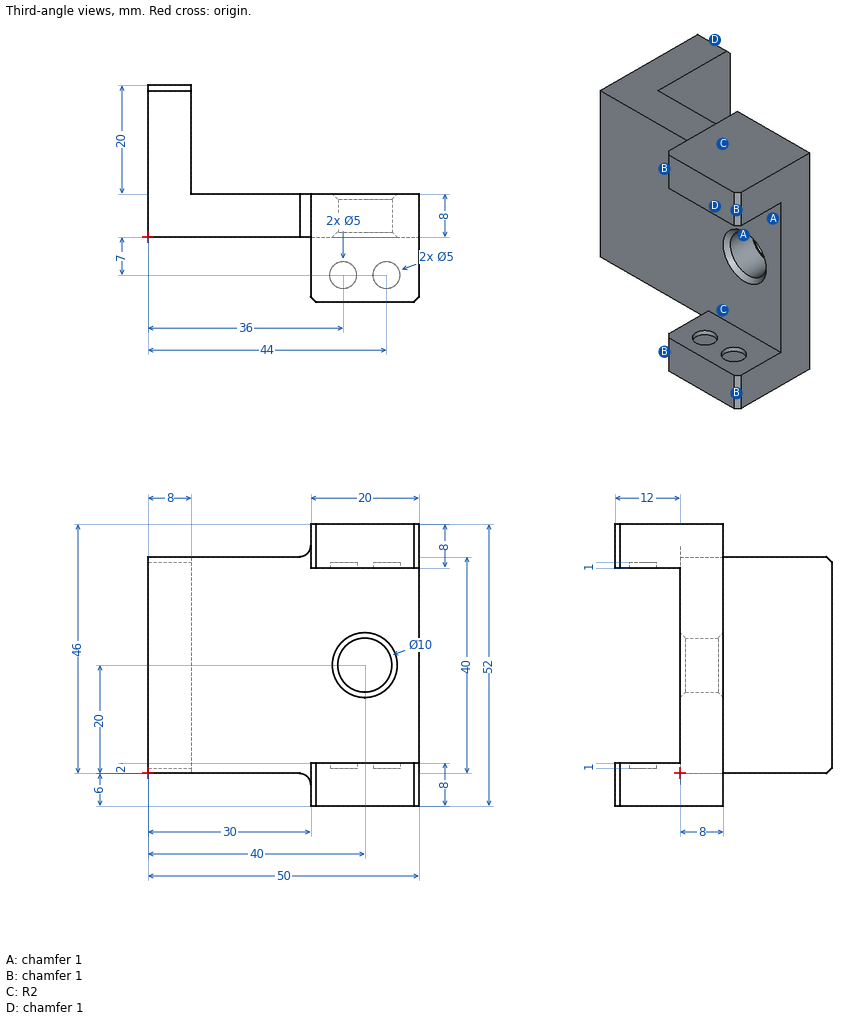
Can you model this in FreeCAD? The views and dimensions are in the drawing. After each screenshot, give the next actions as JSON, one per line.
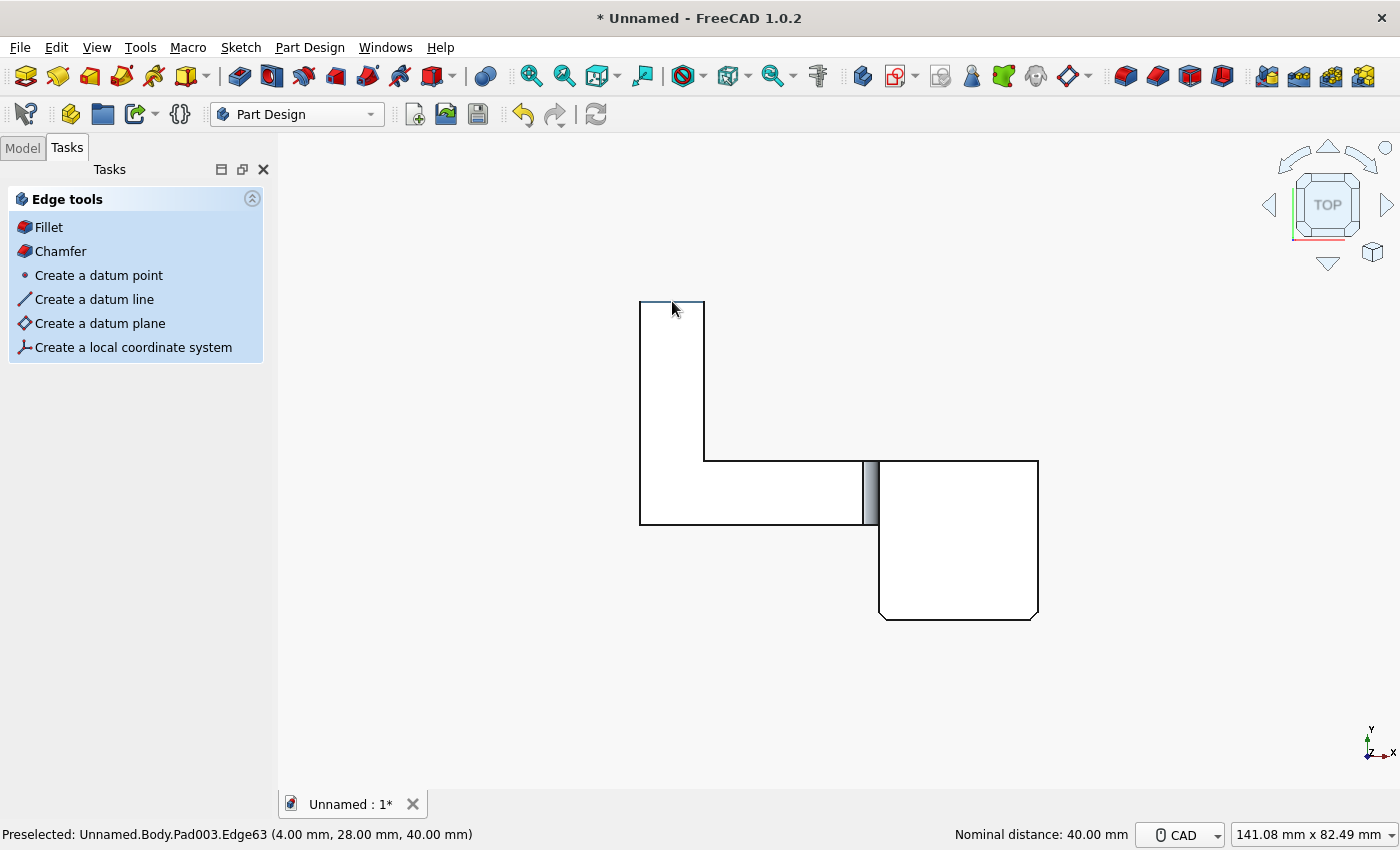
{"action": "left_click", "coordinate": [1158, 76]}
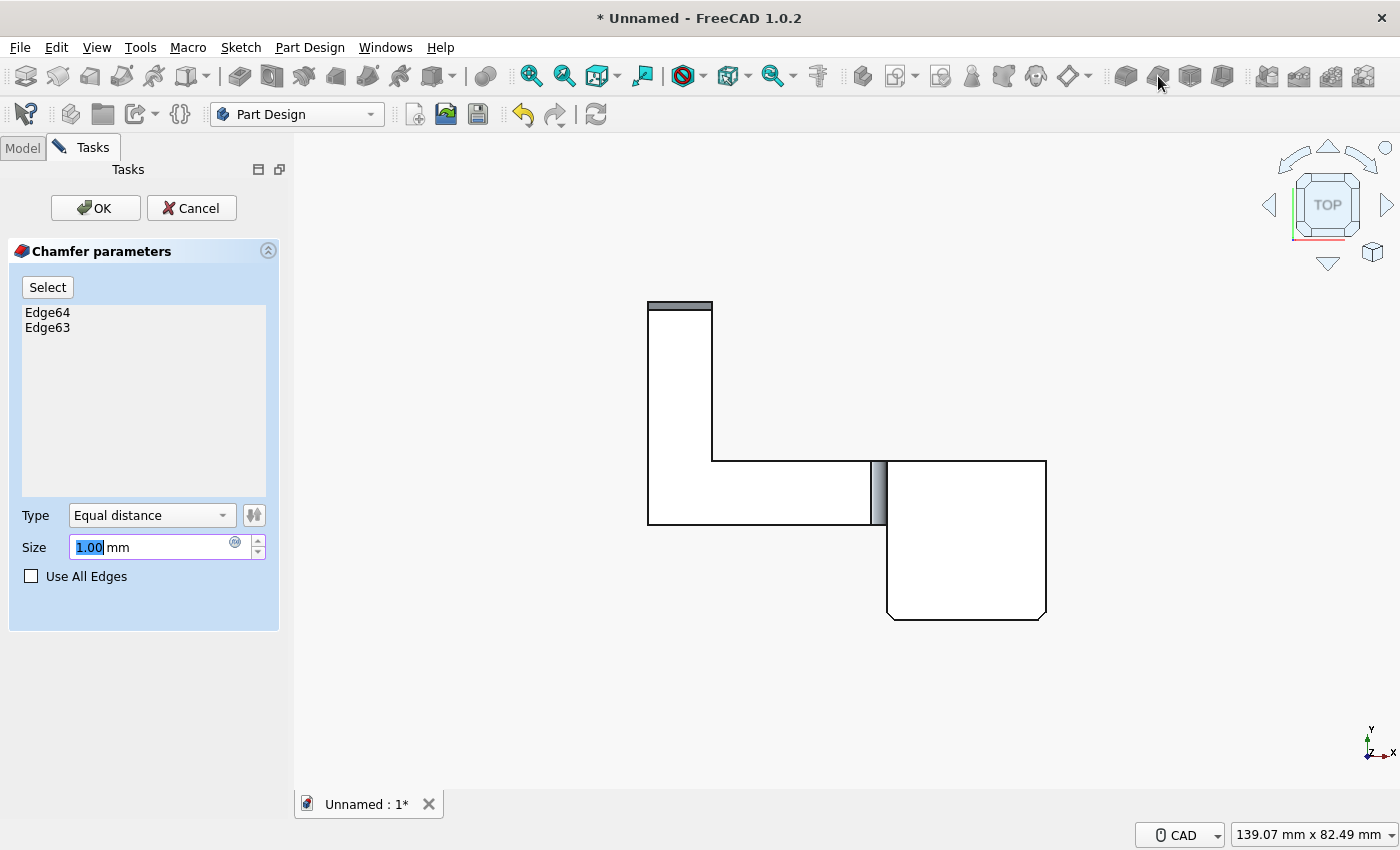
{"action": "type", "text": "1"}
{"action": "key", "text": "Tab"}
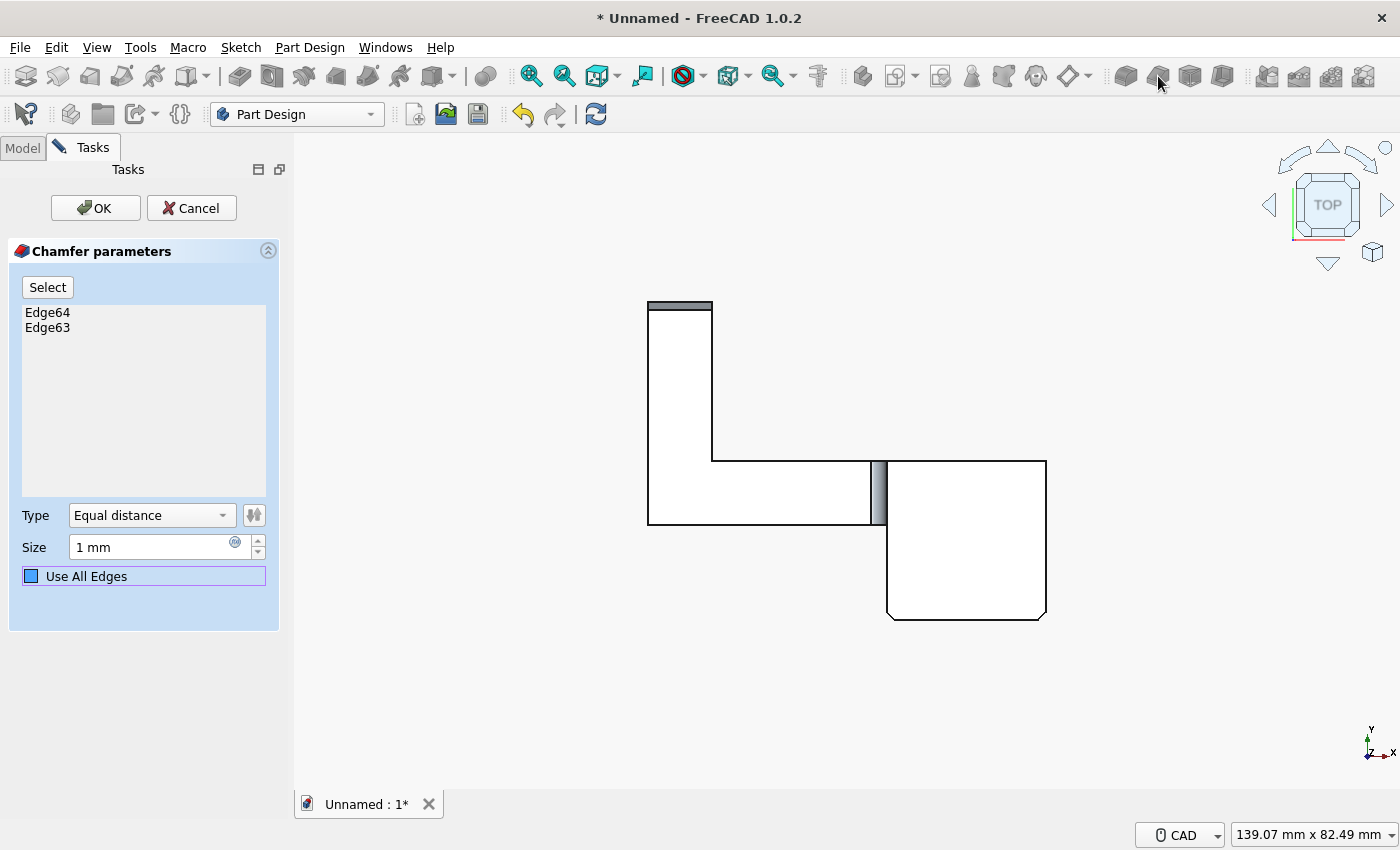
{"action": "left_click", "coordinate": [96, 208]}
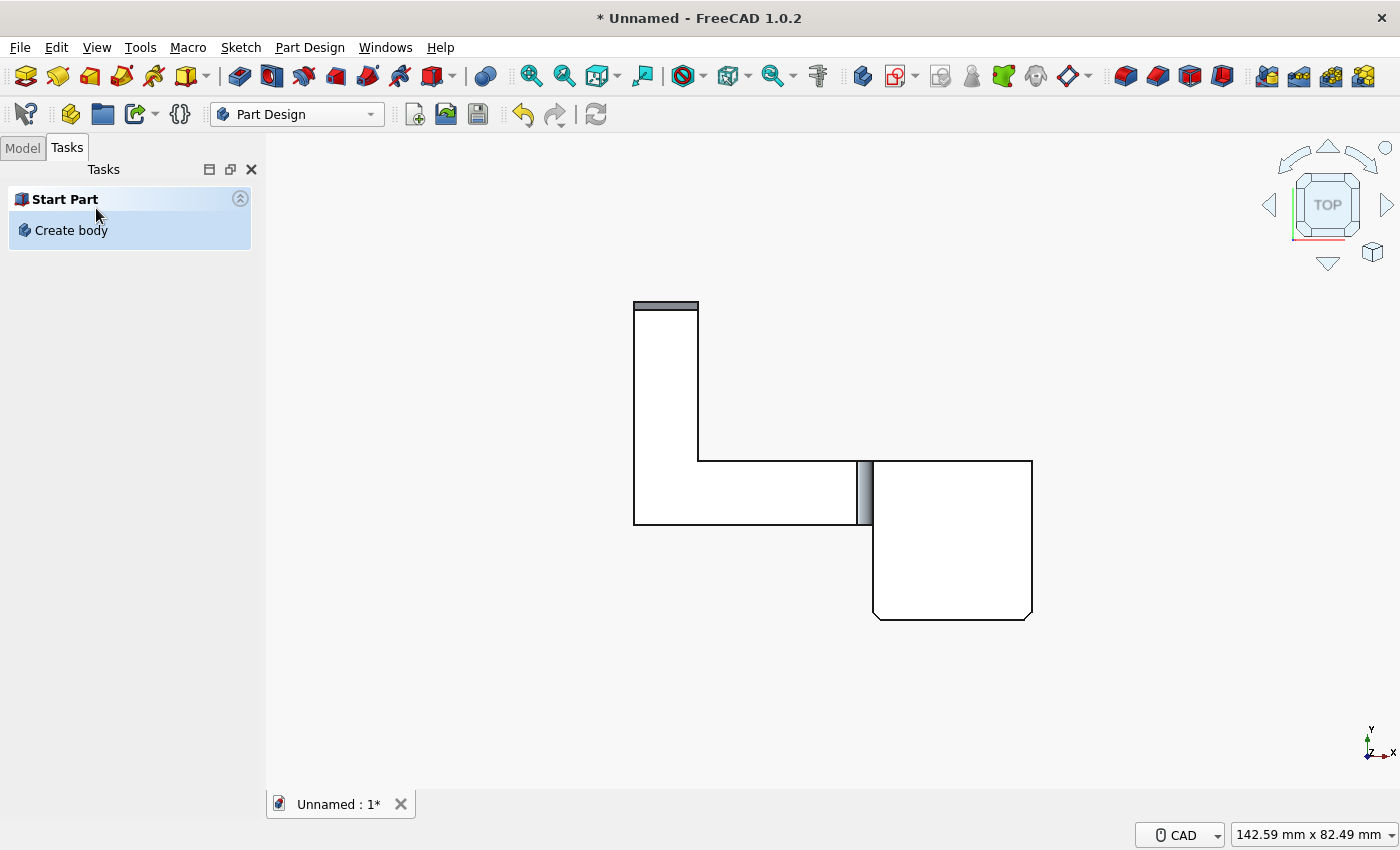
{"action": "left_click", "coordinate": [23, 147]}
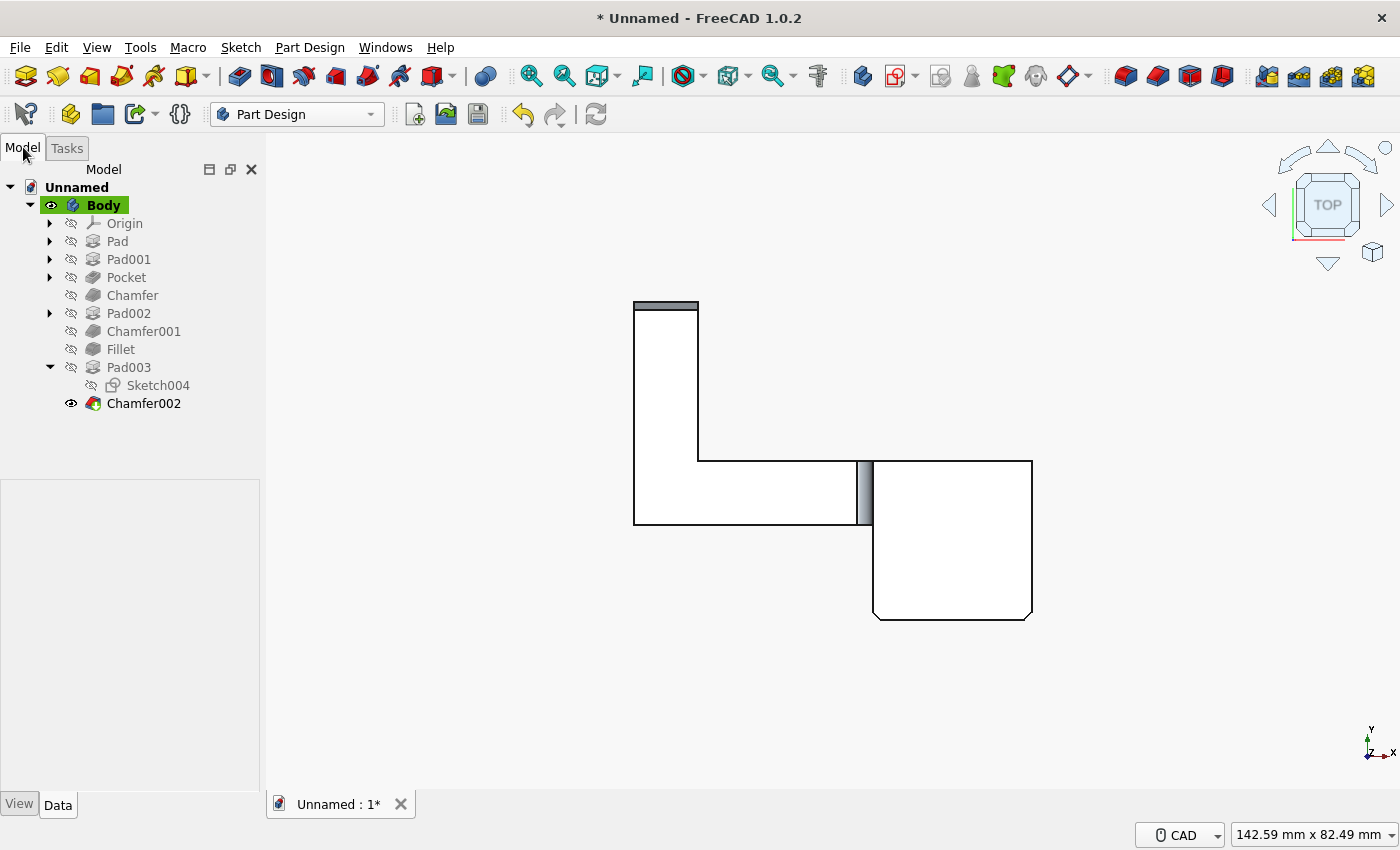
{"action": "left_click", "coordinate": [50, 223]}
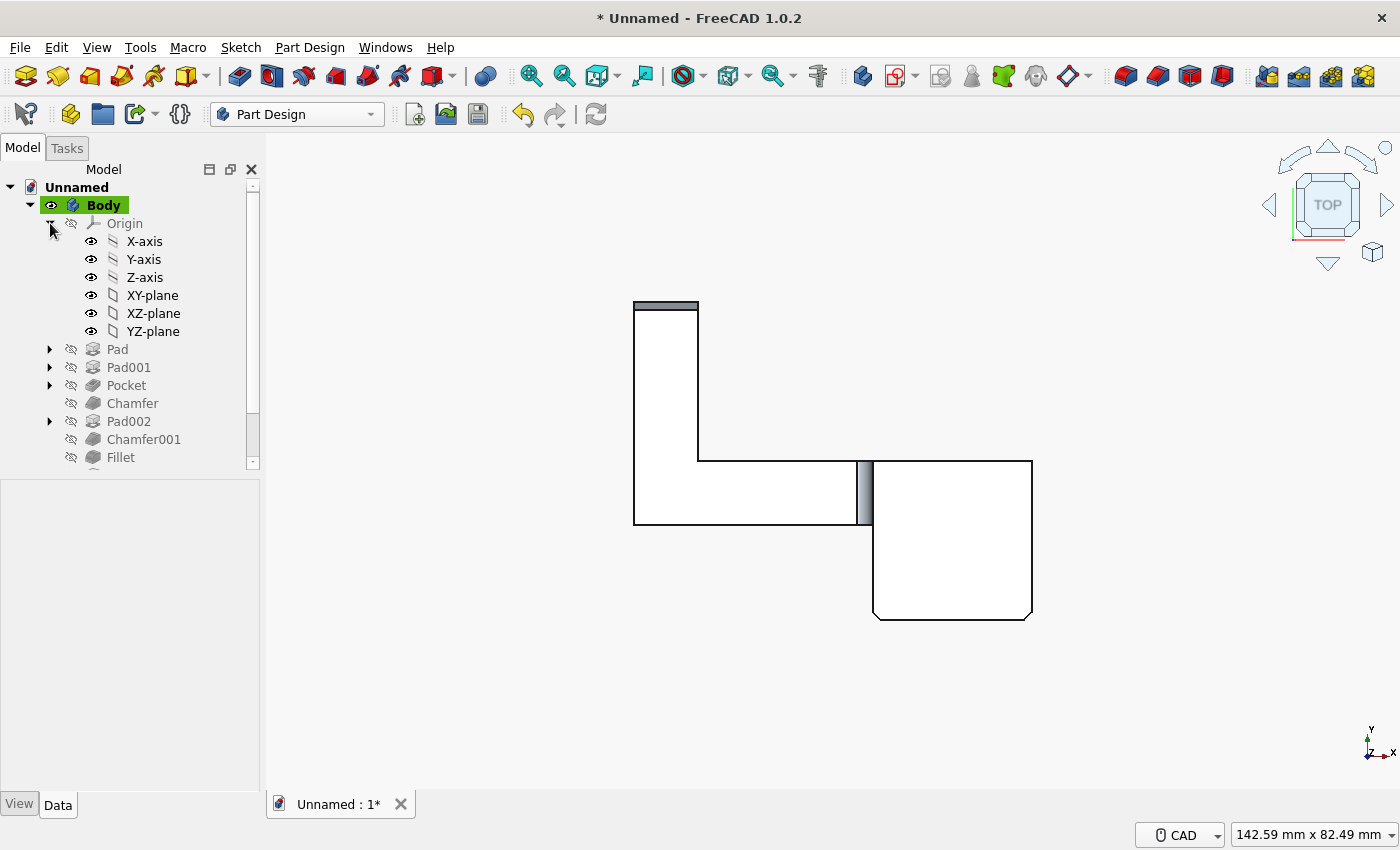
{"action": "left_click", "coordinate": [136, 295]}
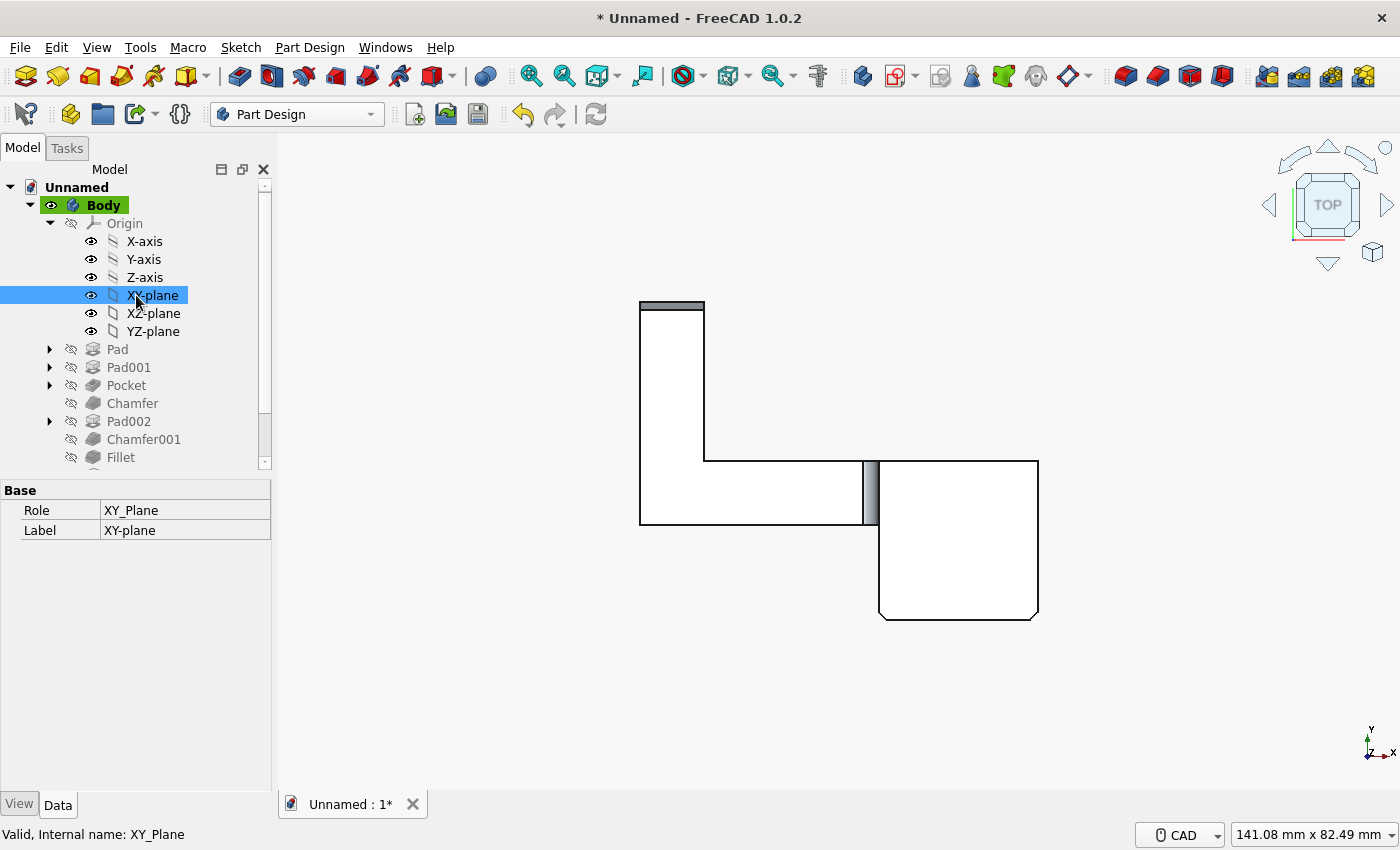
{"action": "left_click", "coordinate": [1068, 76]}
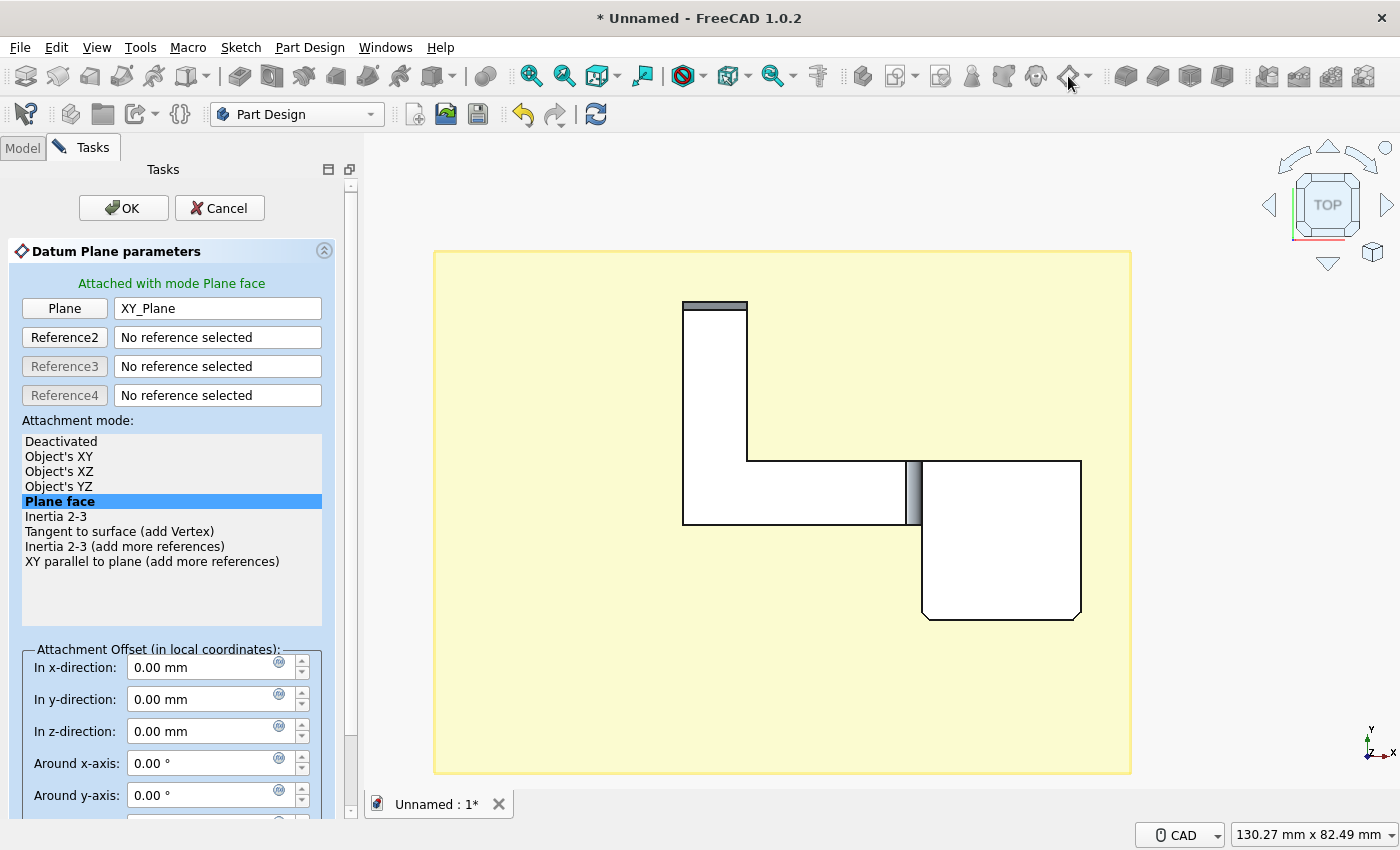
{"action": "triple_click", "coordinate": [210, 731]}